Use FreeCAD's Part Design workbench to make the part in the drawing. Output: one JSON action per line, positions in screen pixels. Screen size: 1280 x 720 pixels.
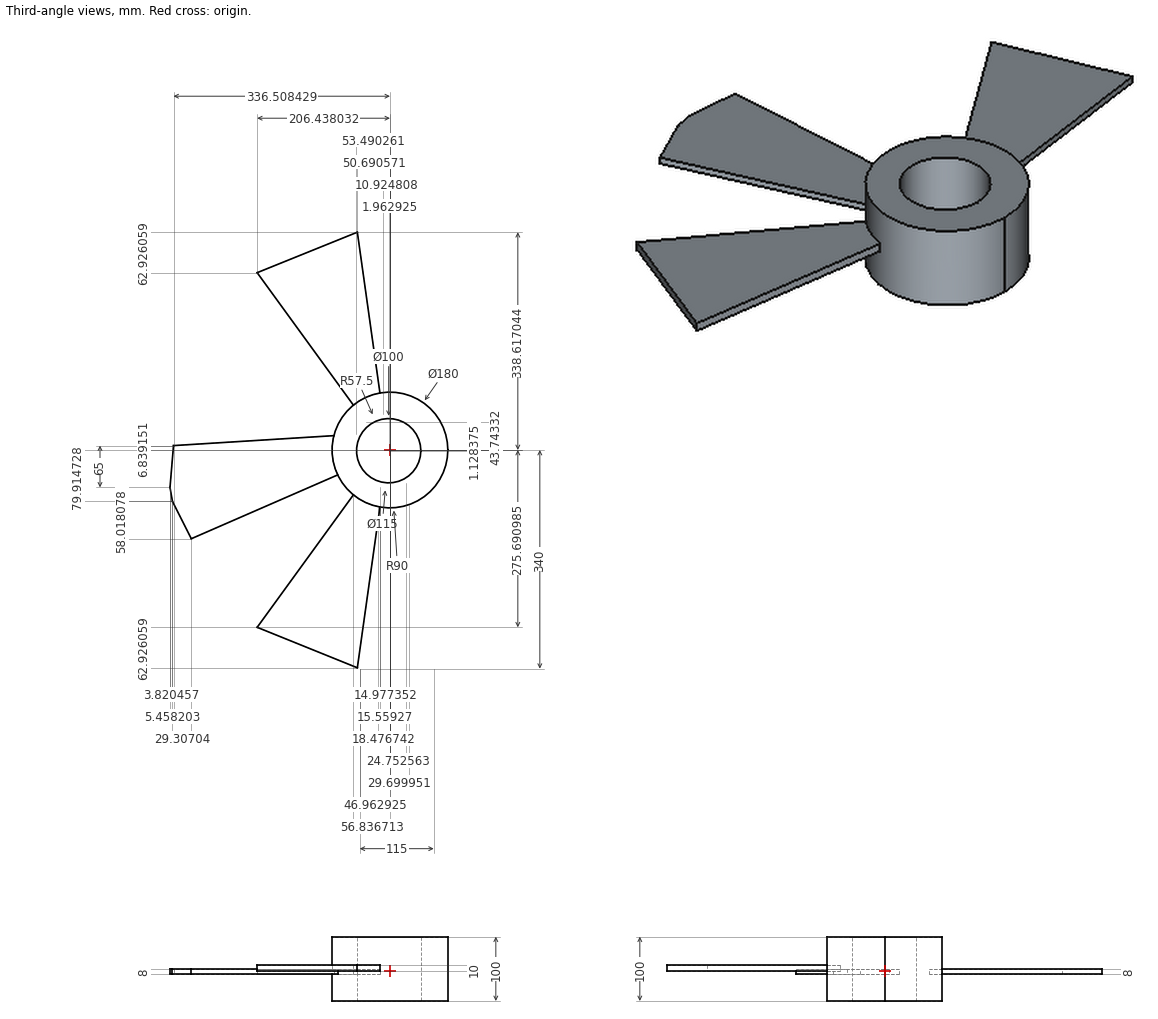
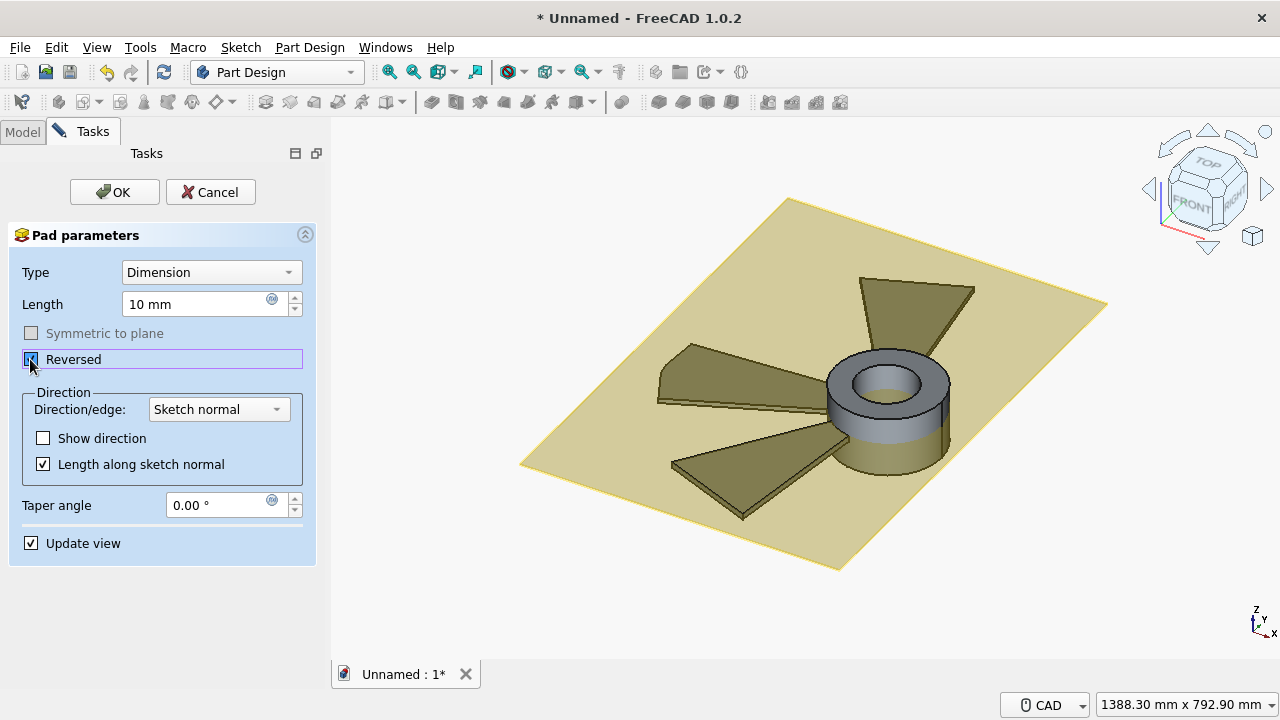
{"action": "left_click", "coordinate": [115, 192]}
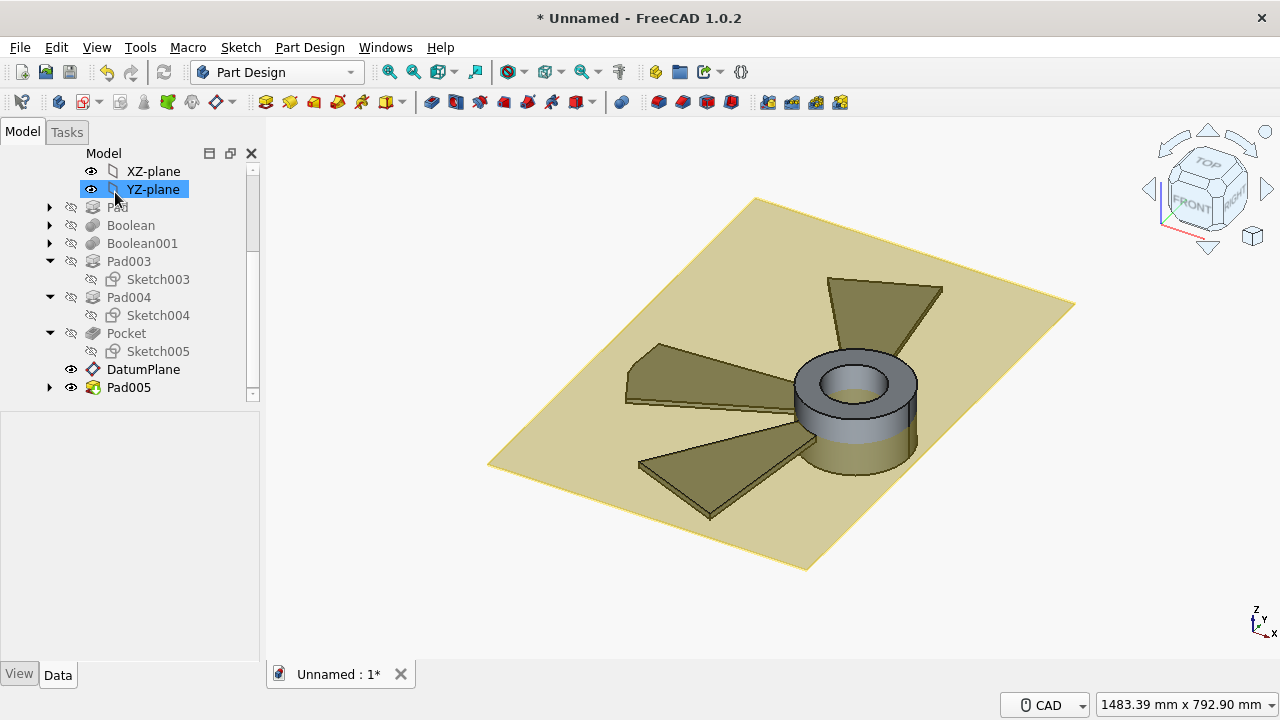
{"action": "left_click", "coordinate": [116, 369]}
{"action": "key", "text": "space"}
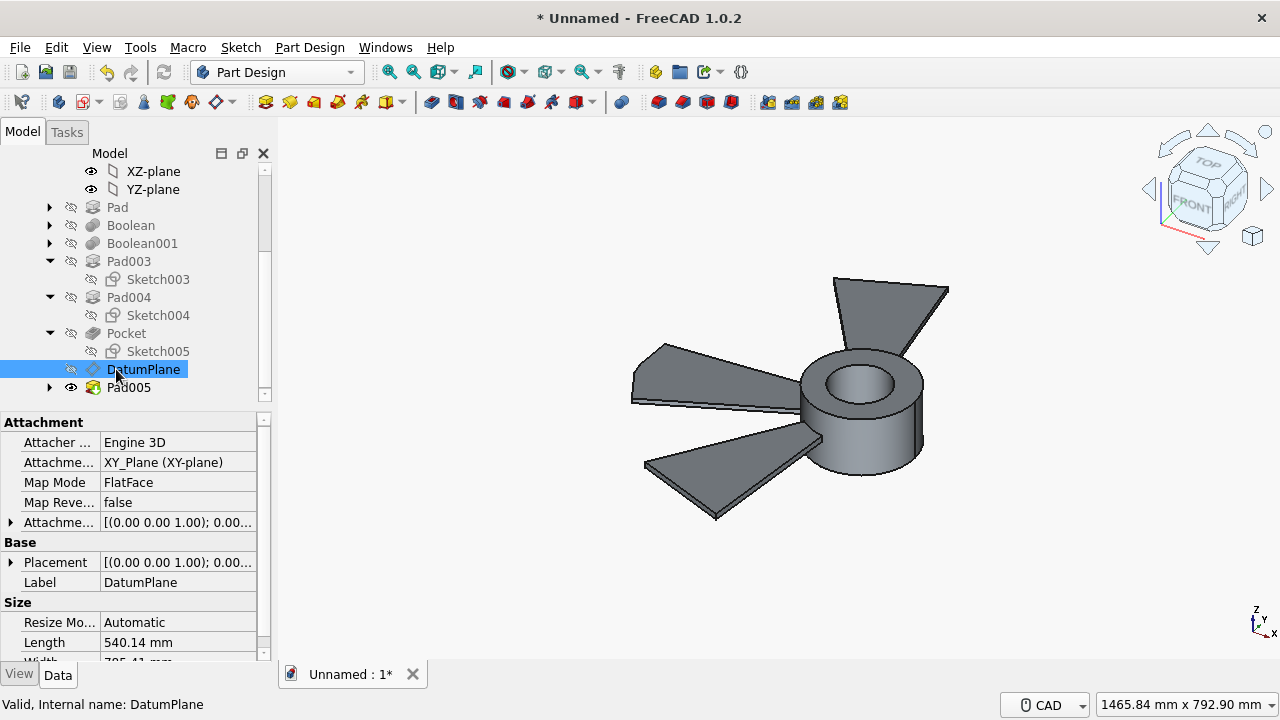
{"action": "key", "text": "0"}